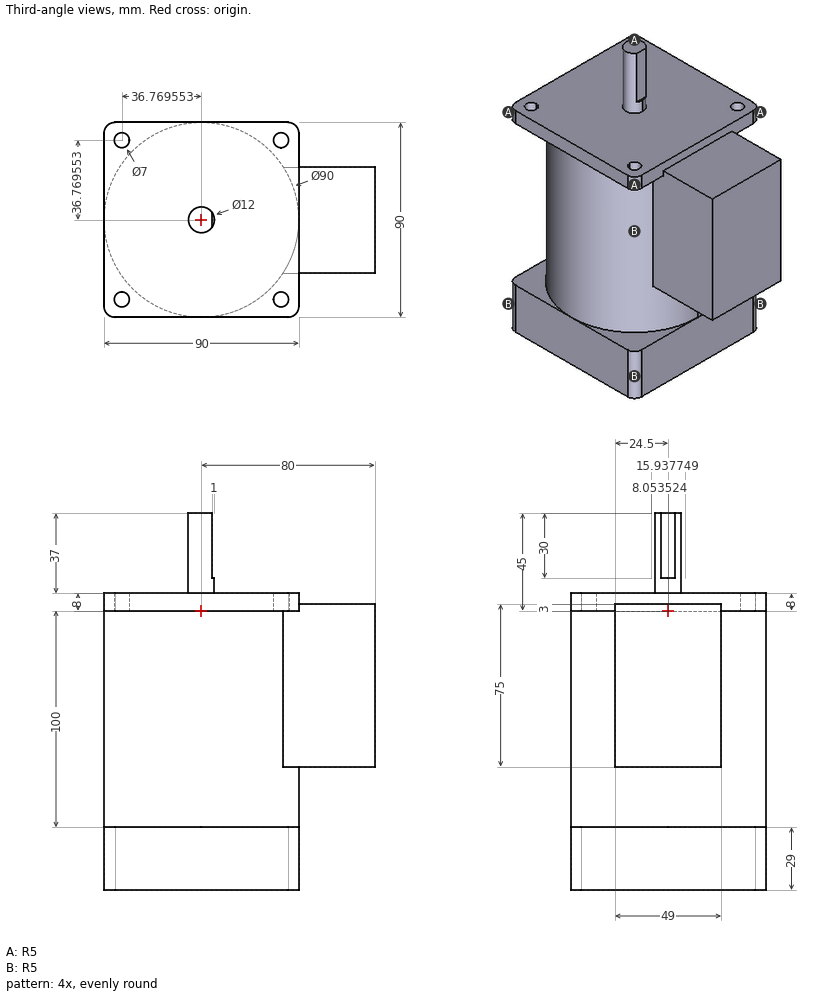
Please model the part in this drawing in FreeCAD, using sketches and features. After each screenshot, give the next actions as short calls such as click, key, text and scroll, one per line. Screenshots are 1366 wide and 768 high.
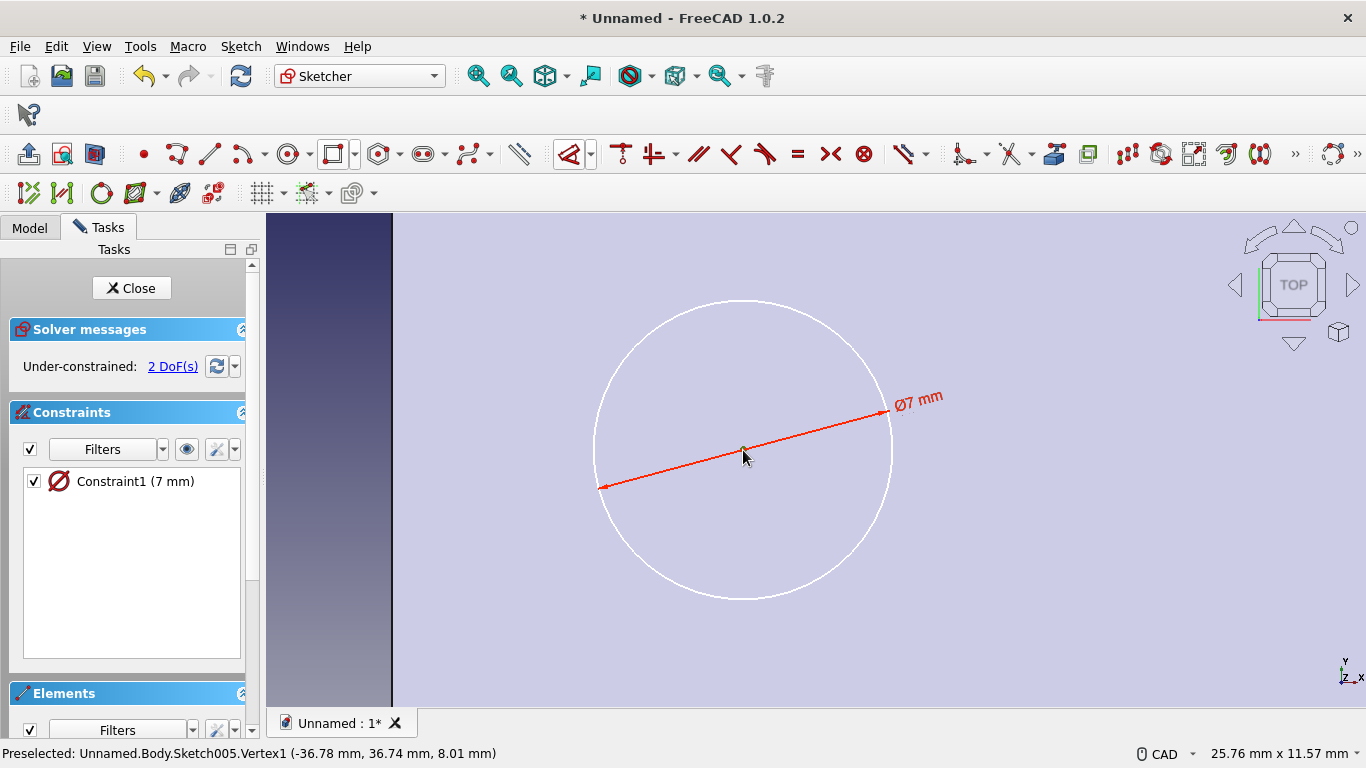
key(l)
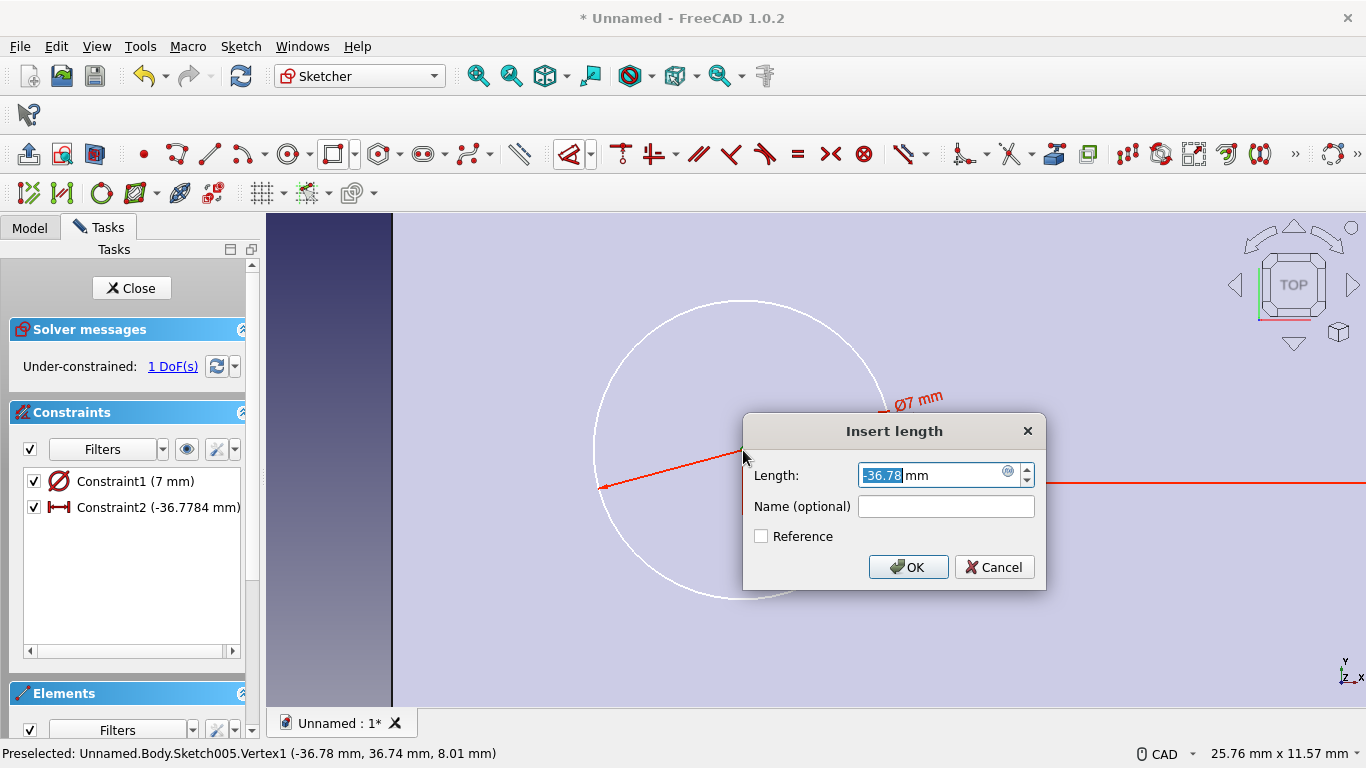
text(-36.769553)
key(Return)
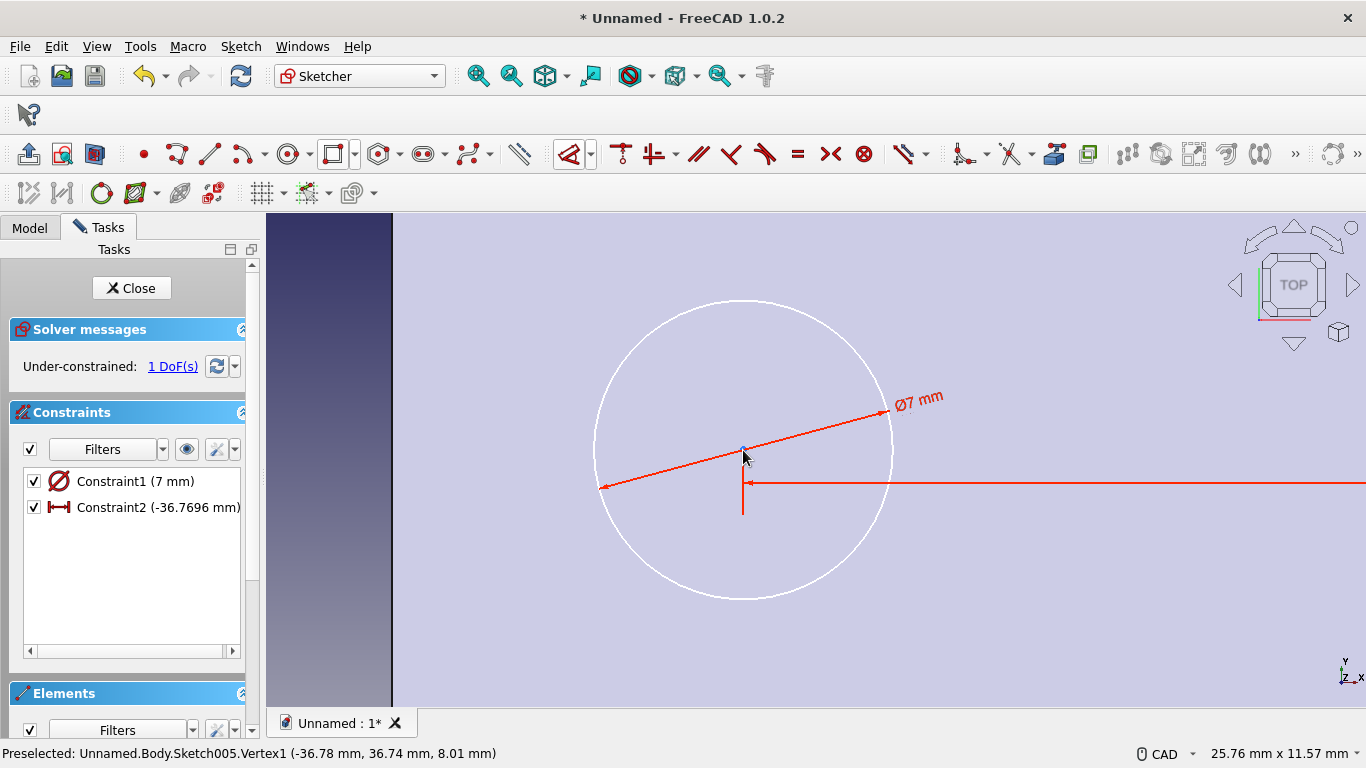
click(743, 450)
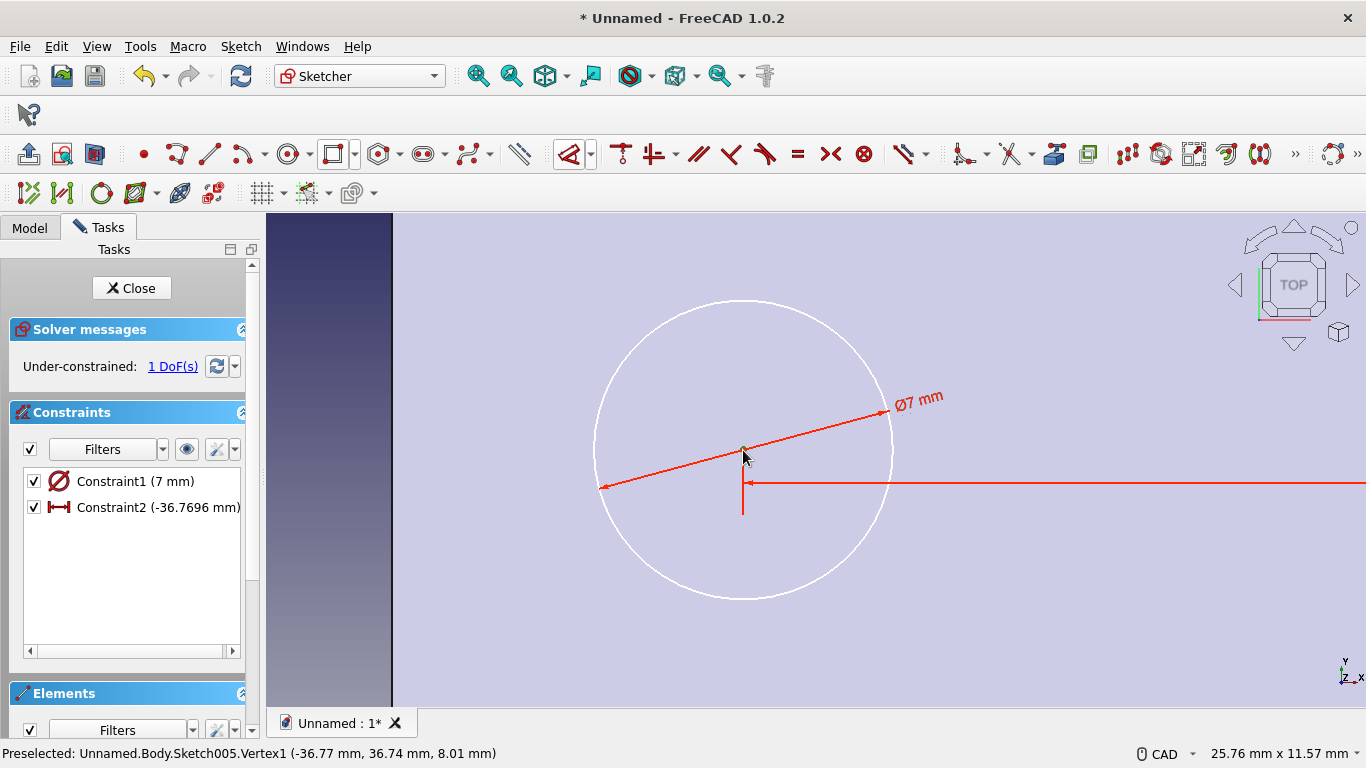
key(i)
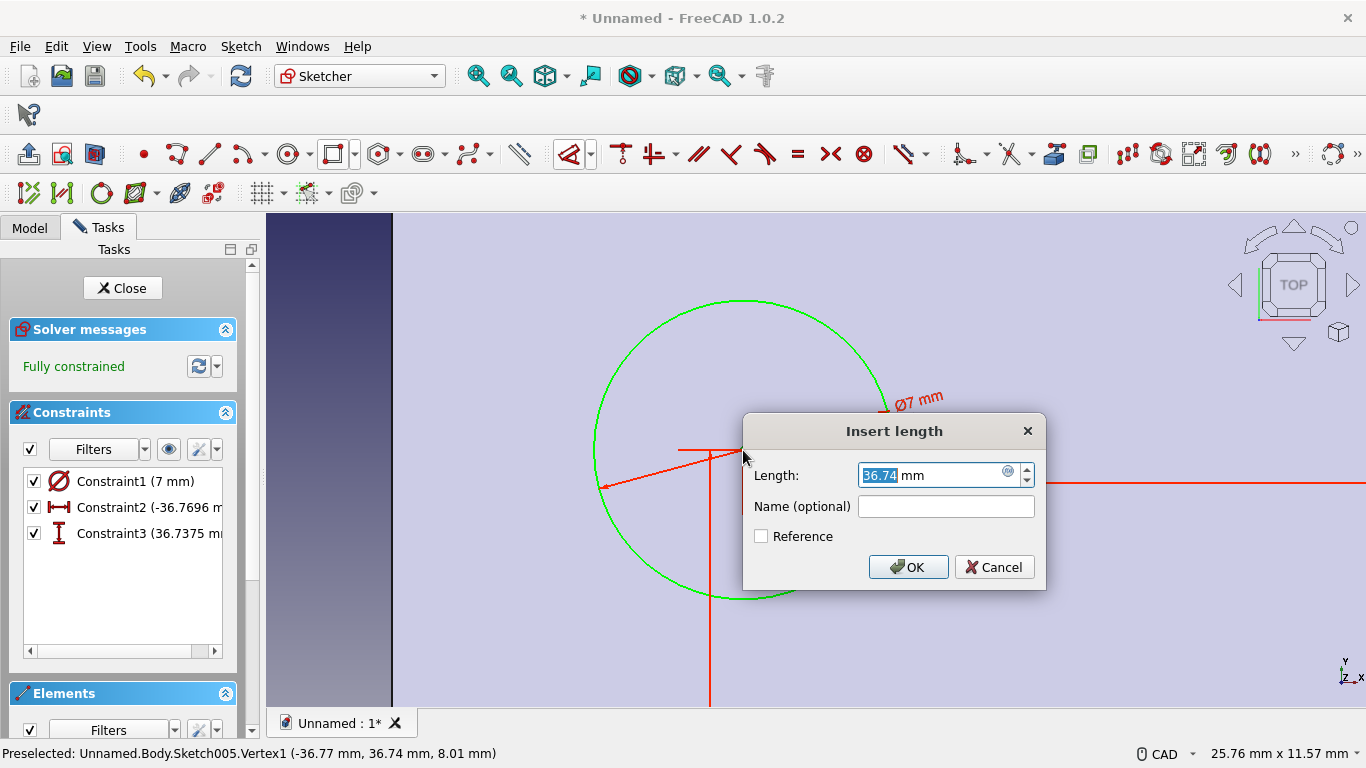
text(36.769553)
key(Return)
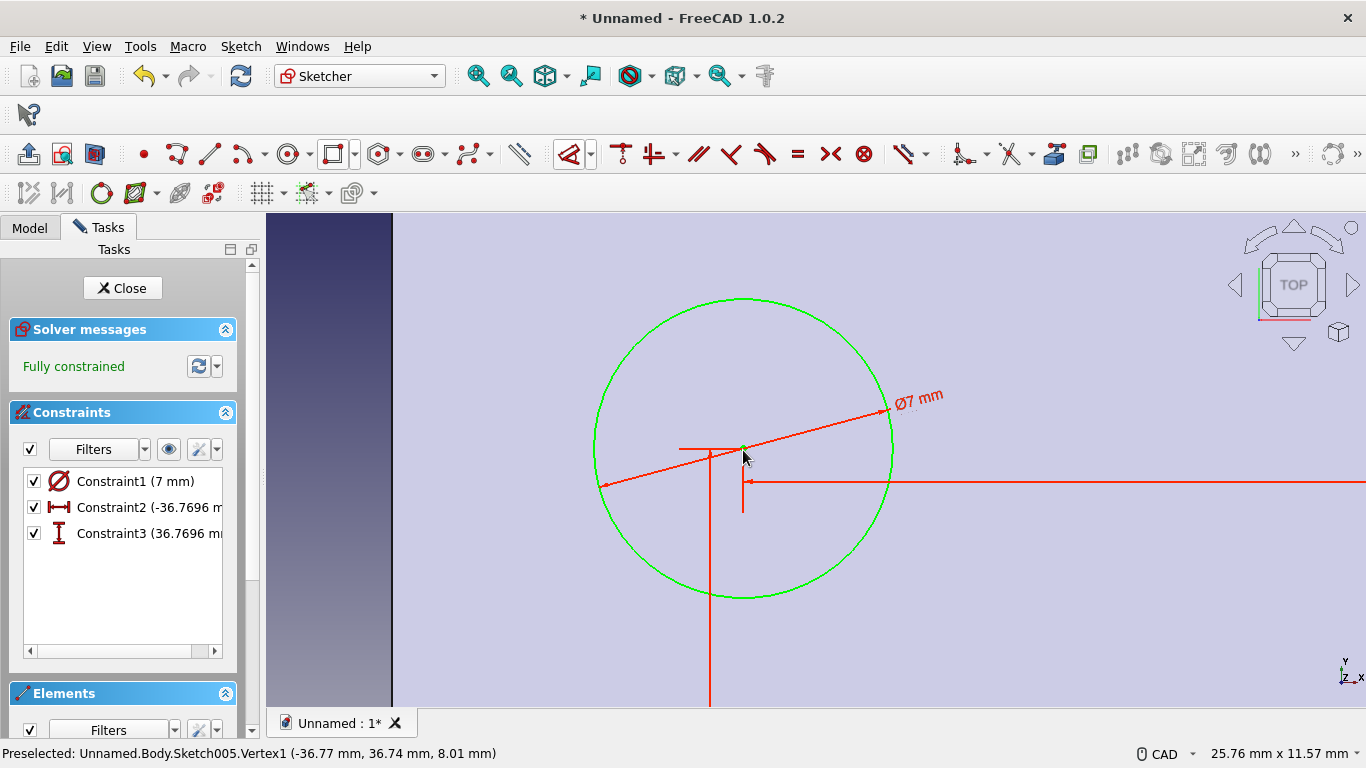
click(123, 288)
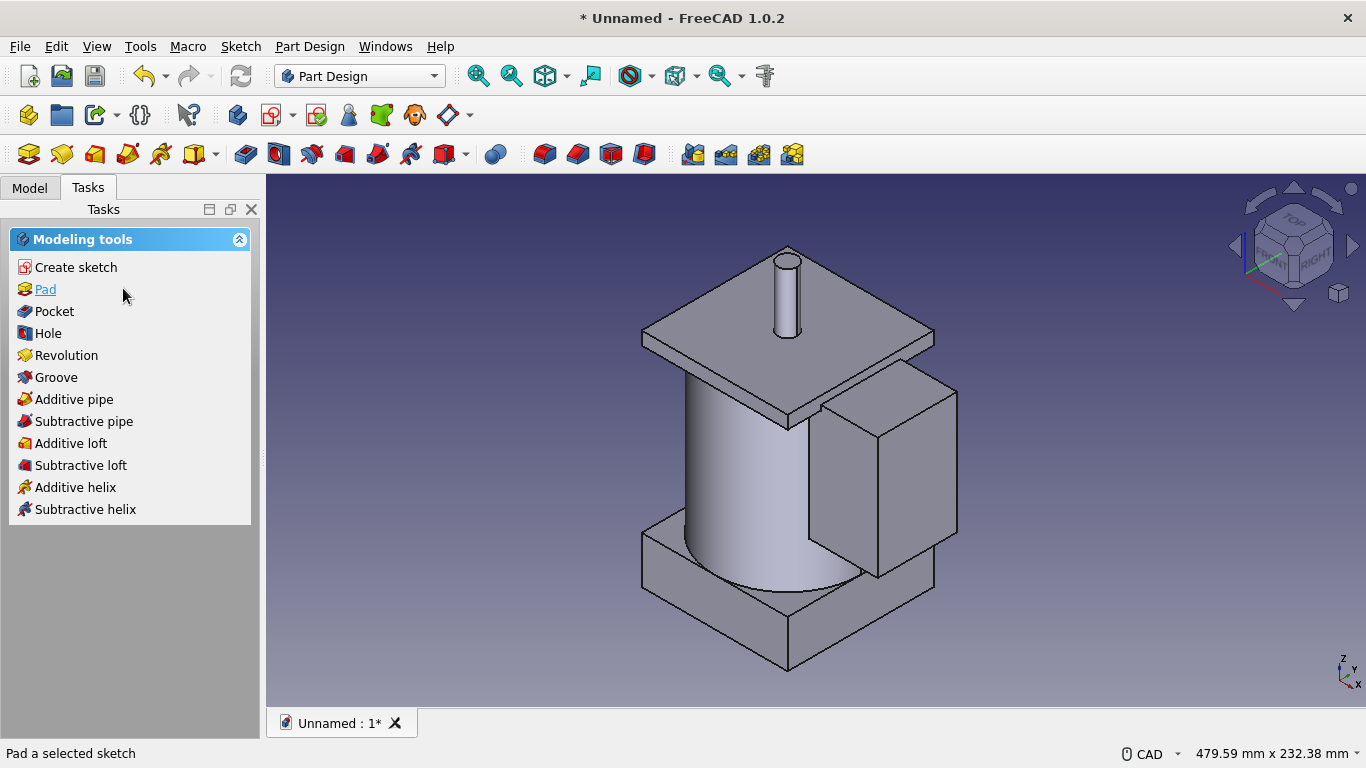
click(246, 154)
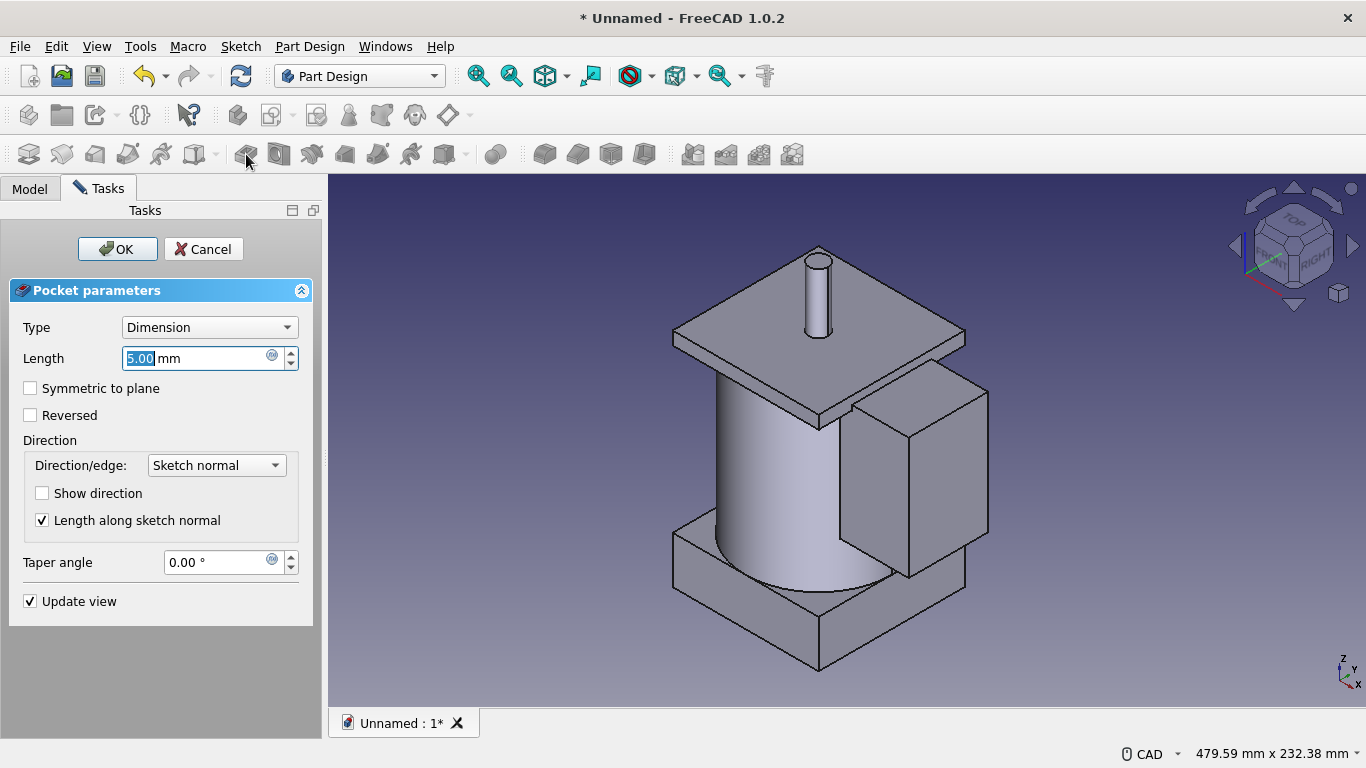
text(8)
key(Tab)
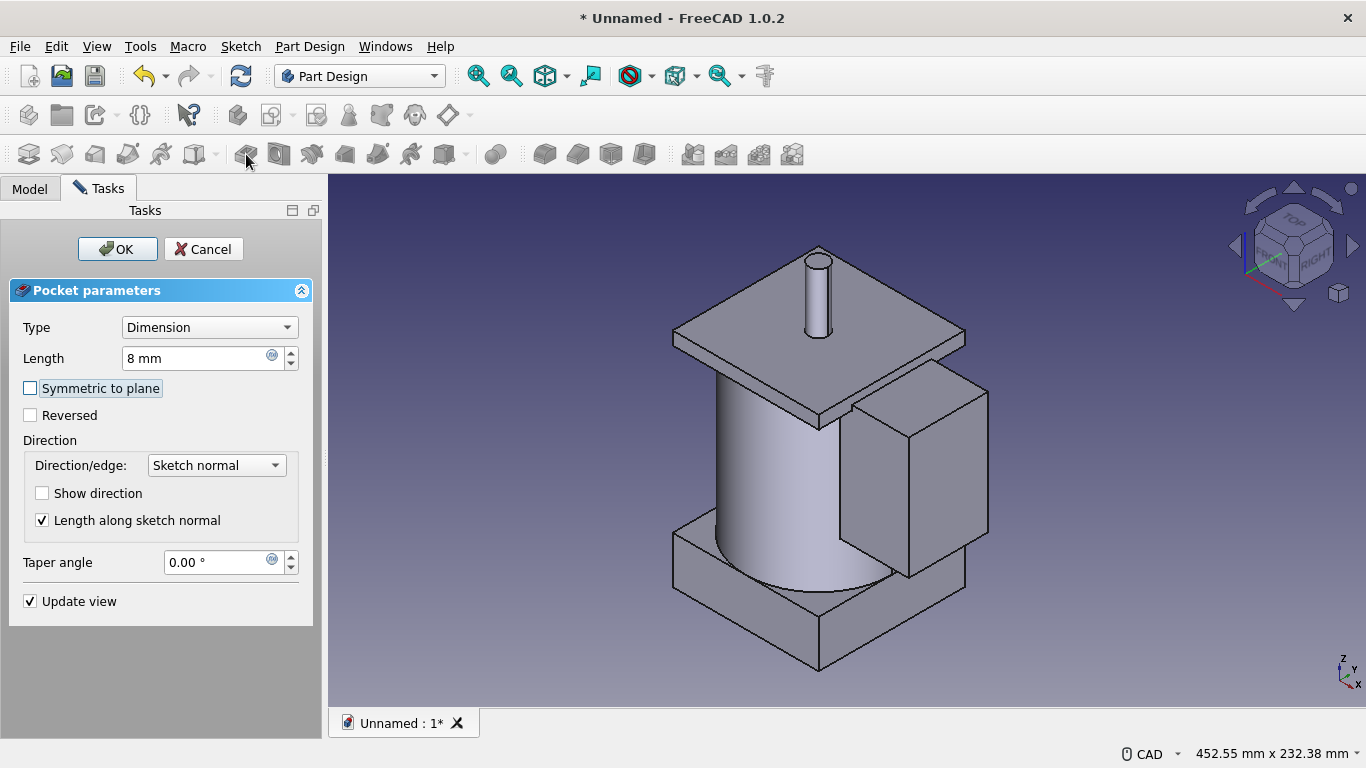
click(118, 249)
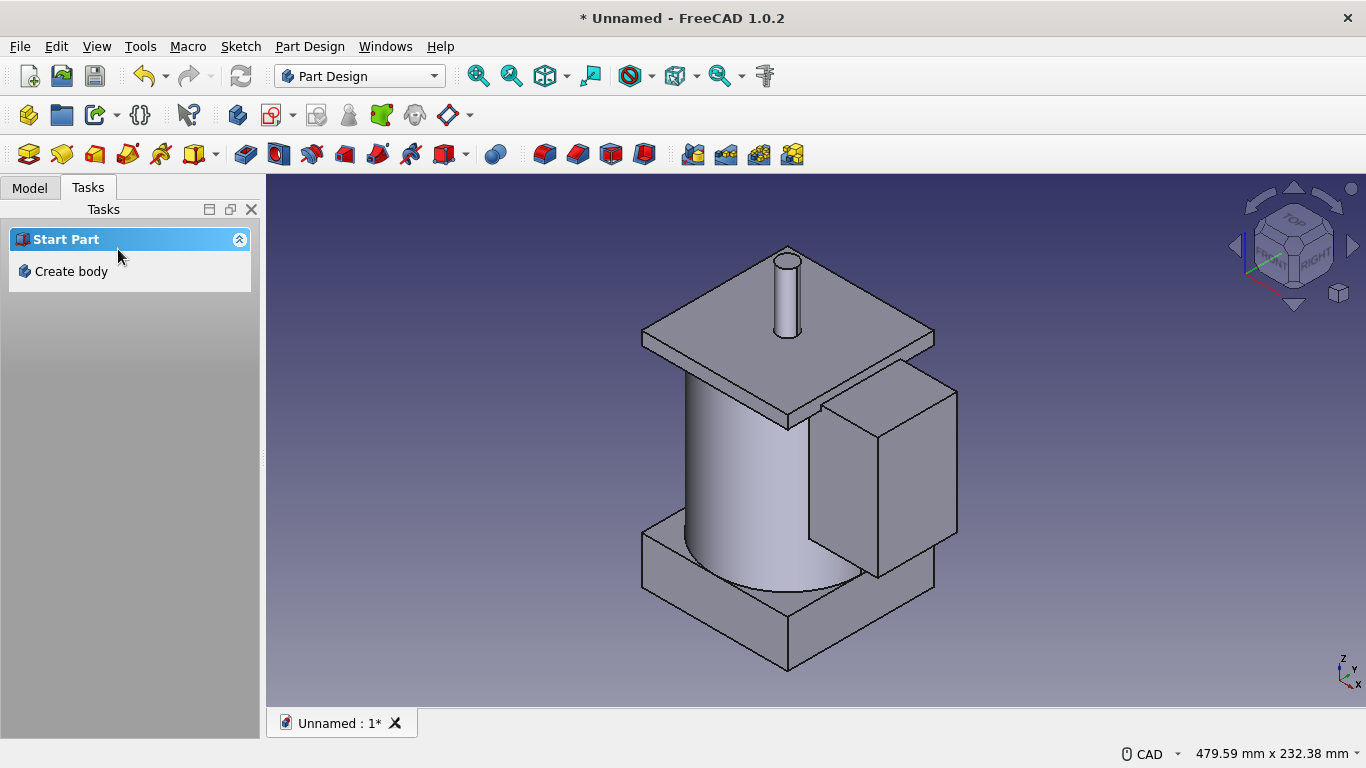
click(788, 421)